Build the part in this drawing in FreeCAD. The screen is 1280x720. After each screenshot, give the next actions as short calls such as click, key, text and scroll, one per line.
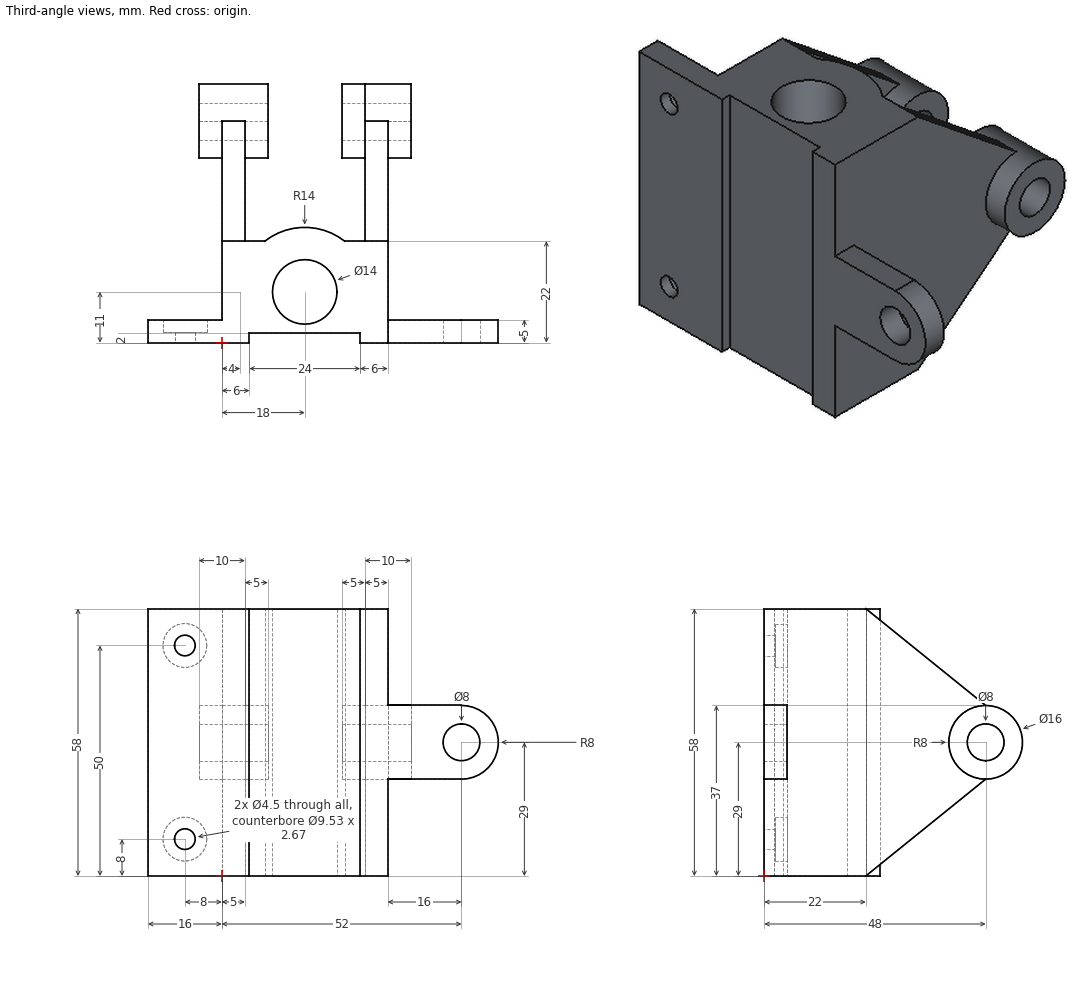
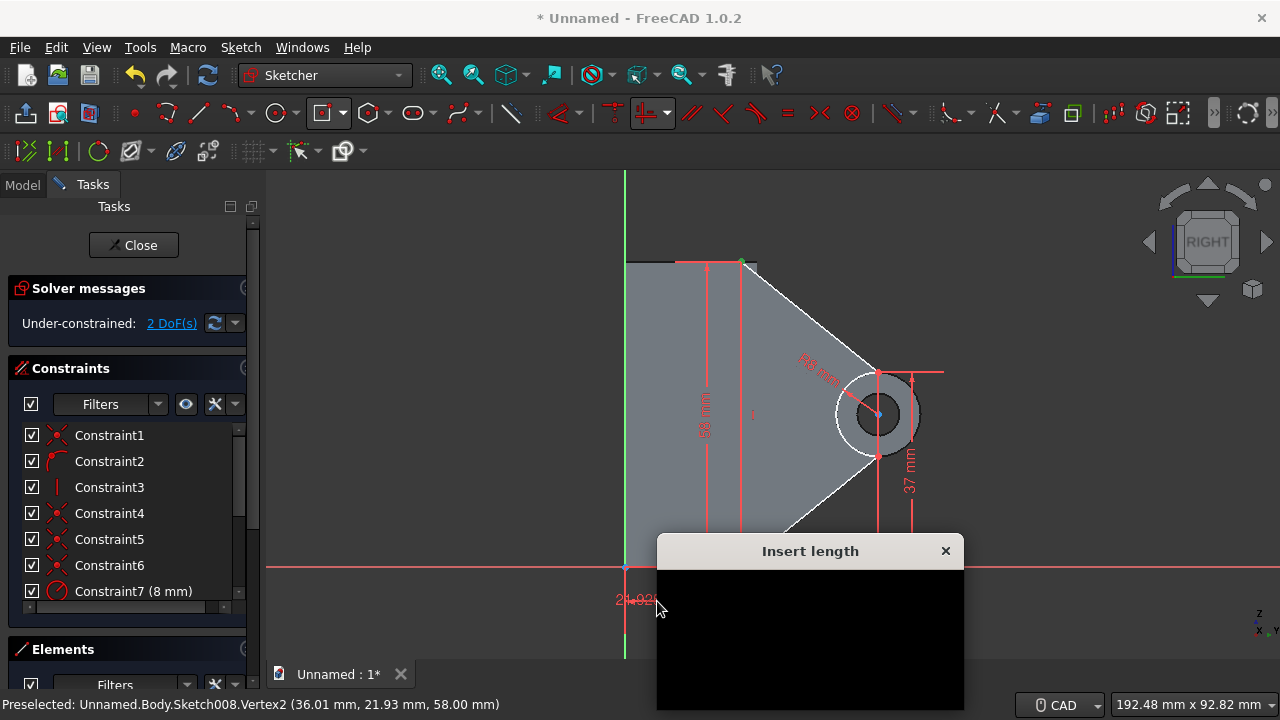
text(22)
key(Return)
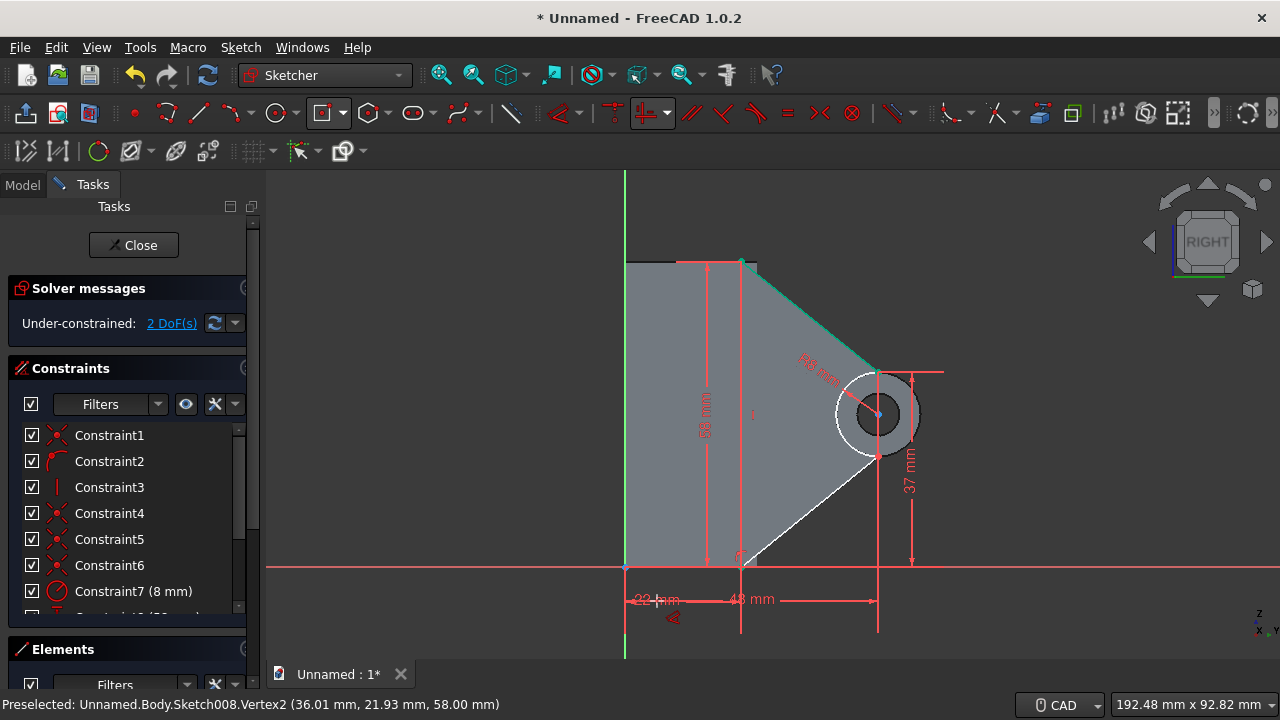
click(878, 457)
click(840, 601)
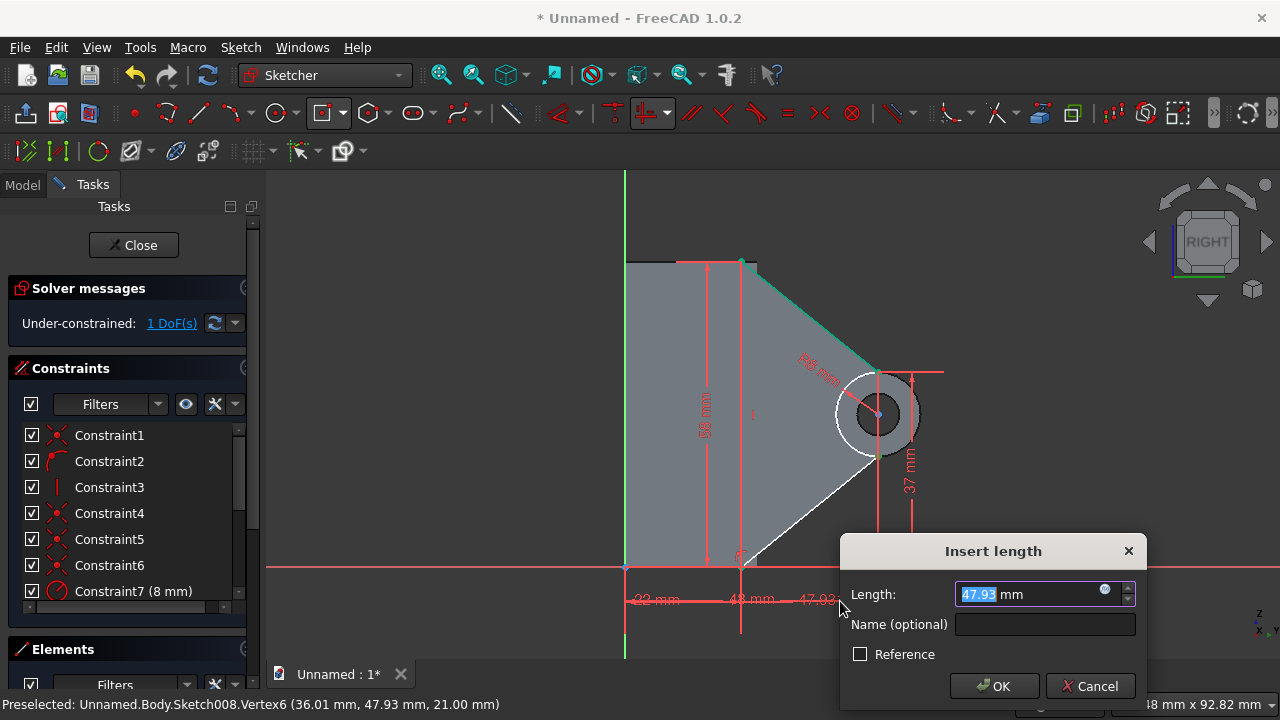
text(48)
key(Return)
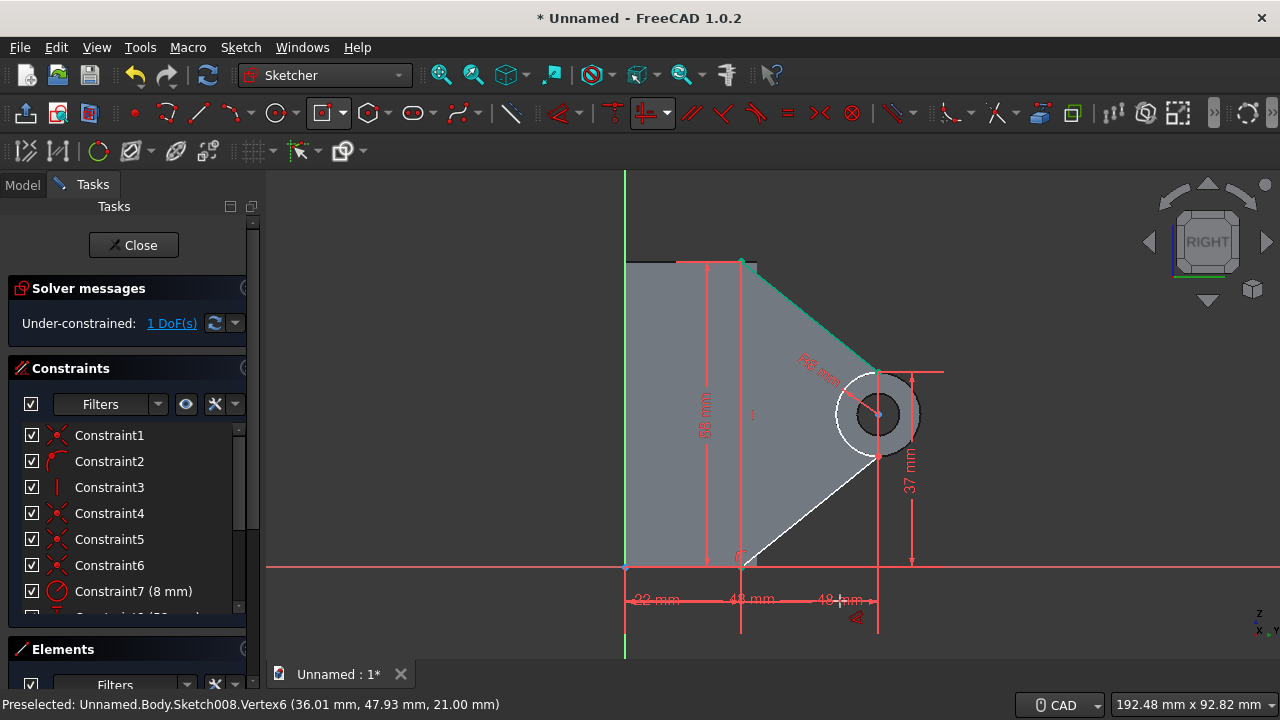
click(878, 414)
click(694, 380)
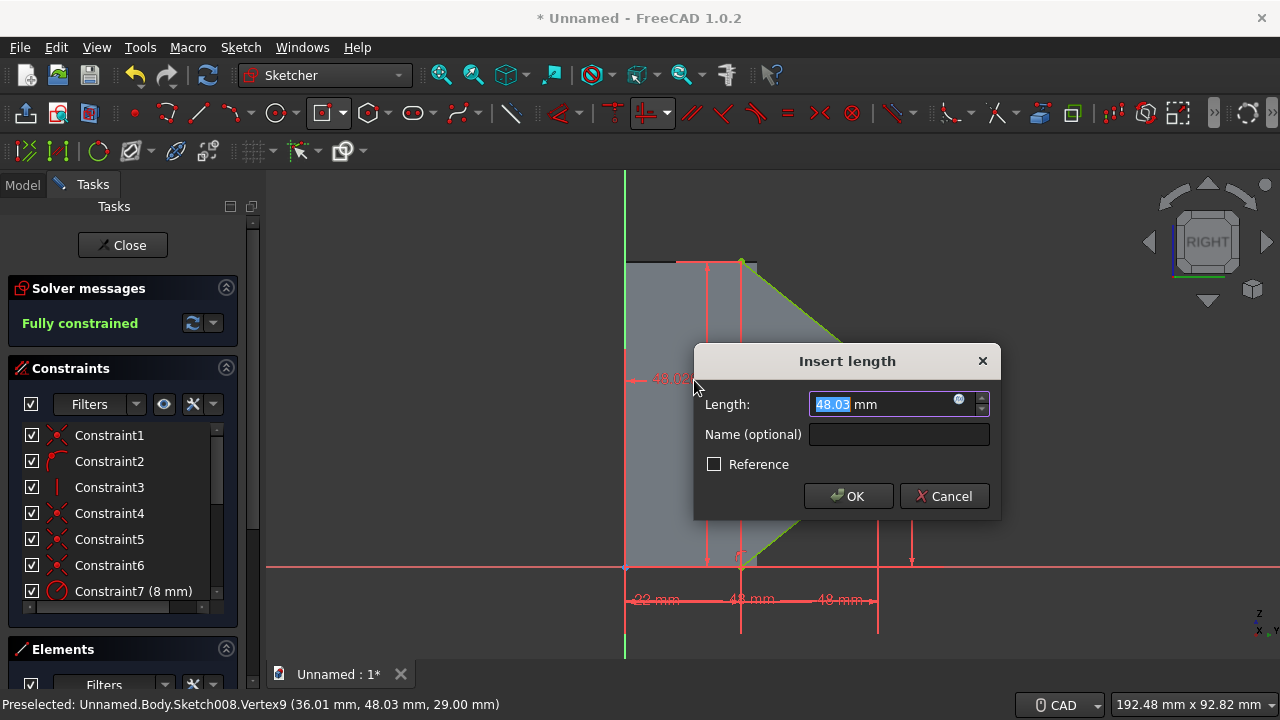
text(48)
key(Return)
key(Escape)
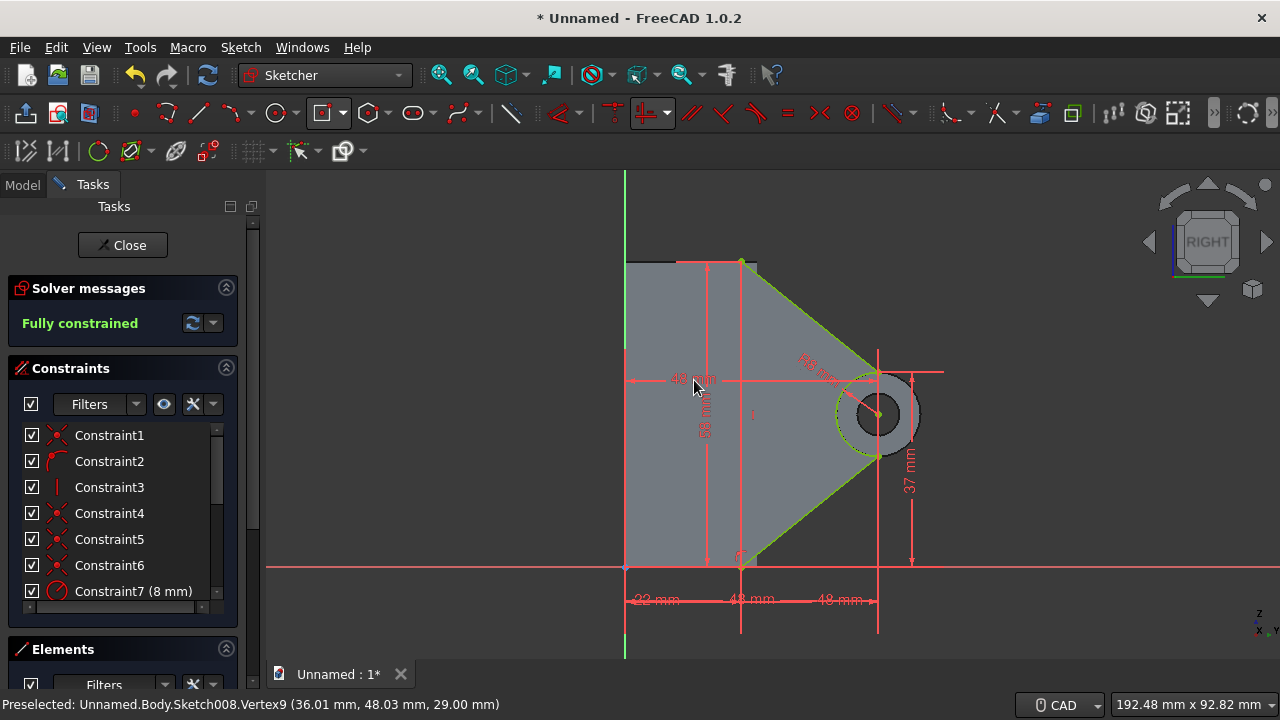
click(123, 245)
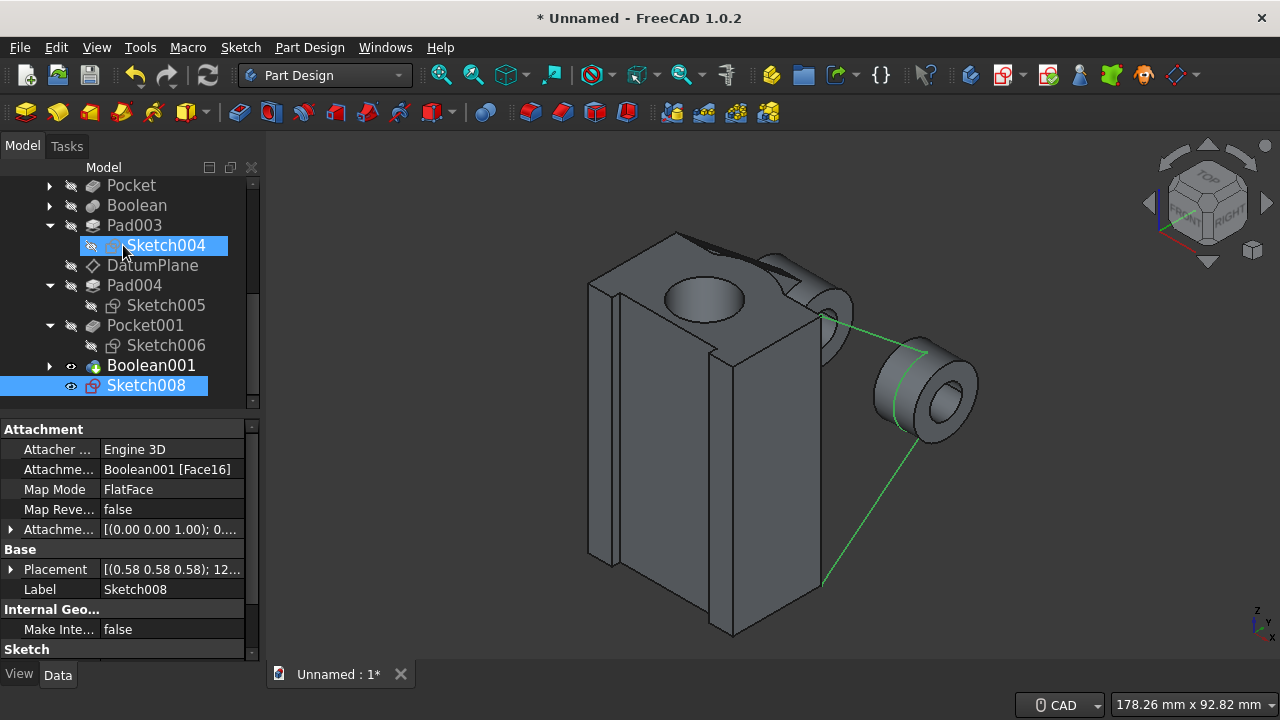
click(26, 112)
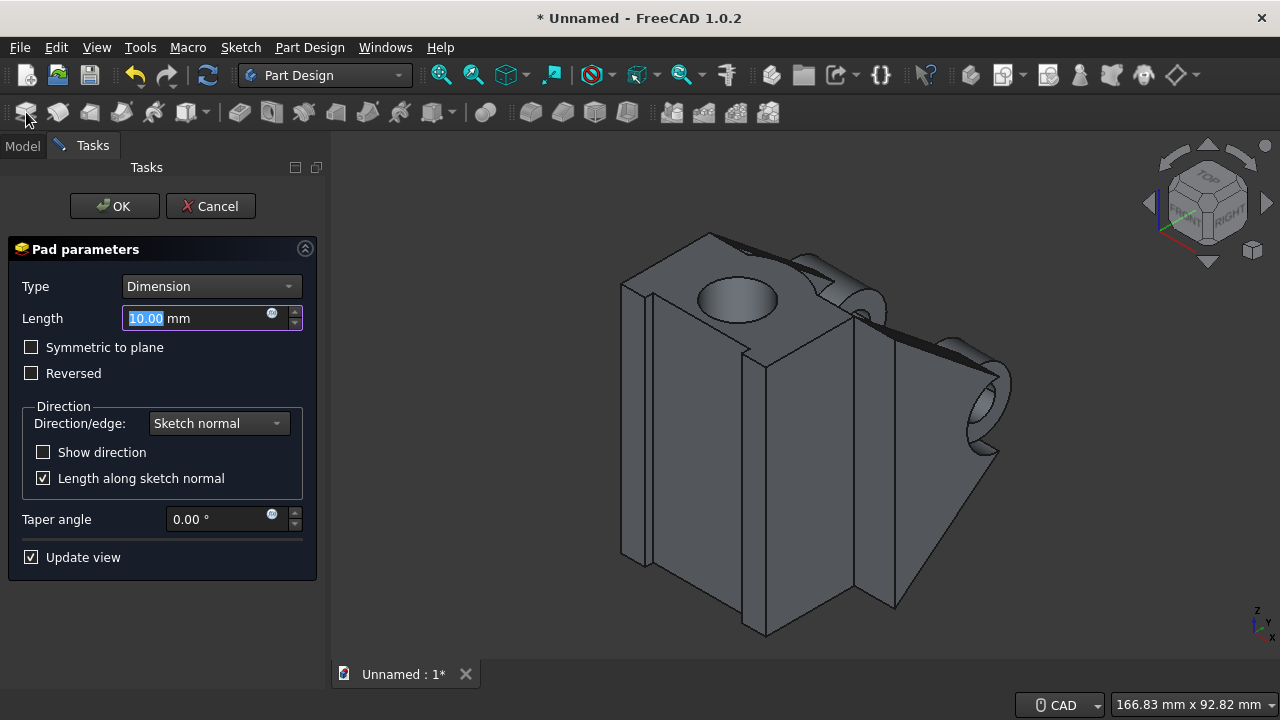
text(5)
key(Tab)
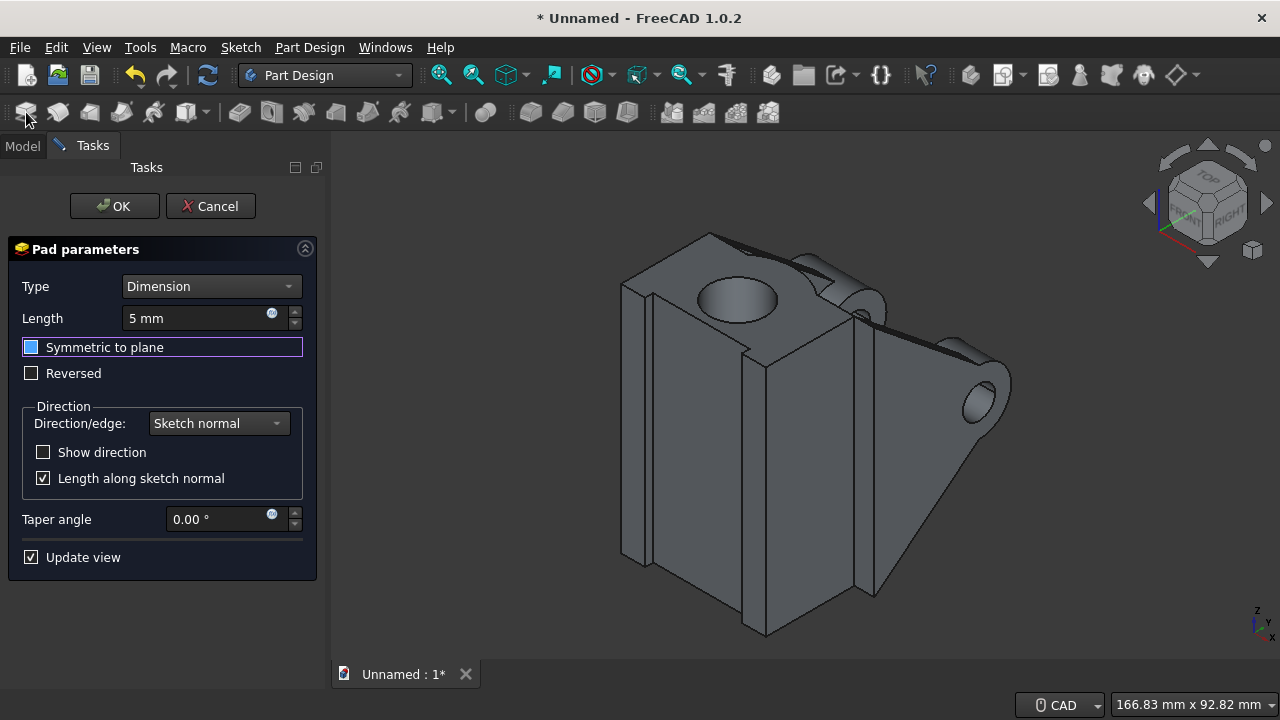
click(30, 373)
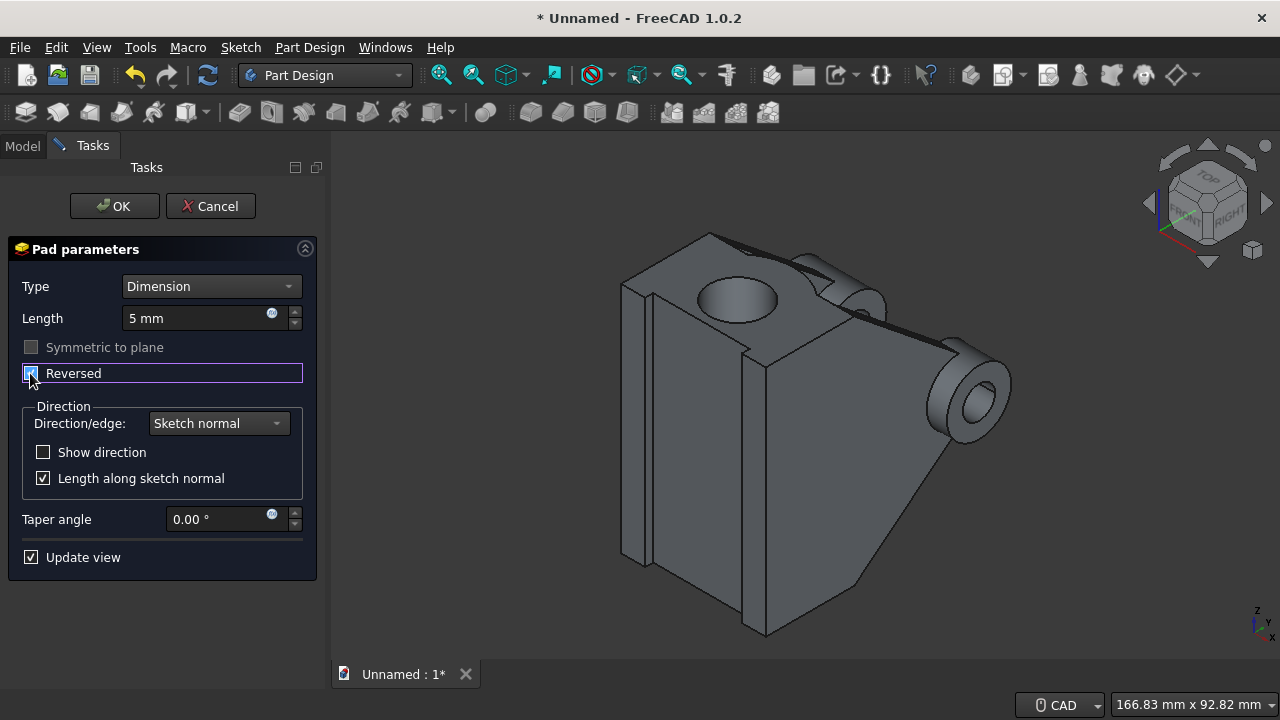
click(115, 206)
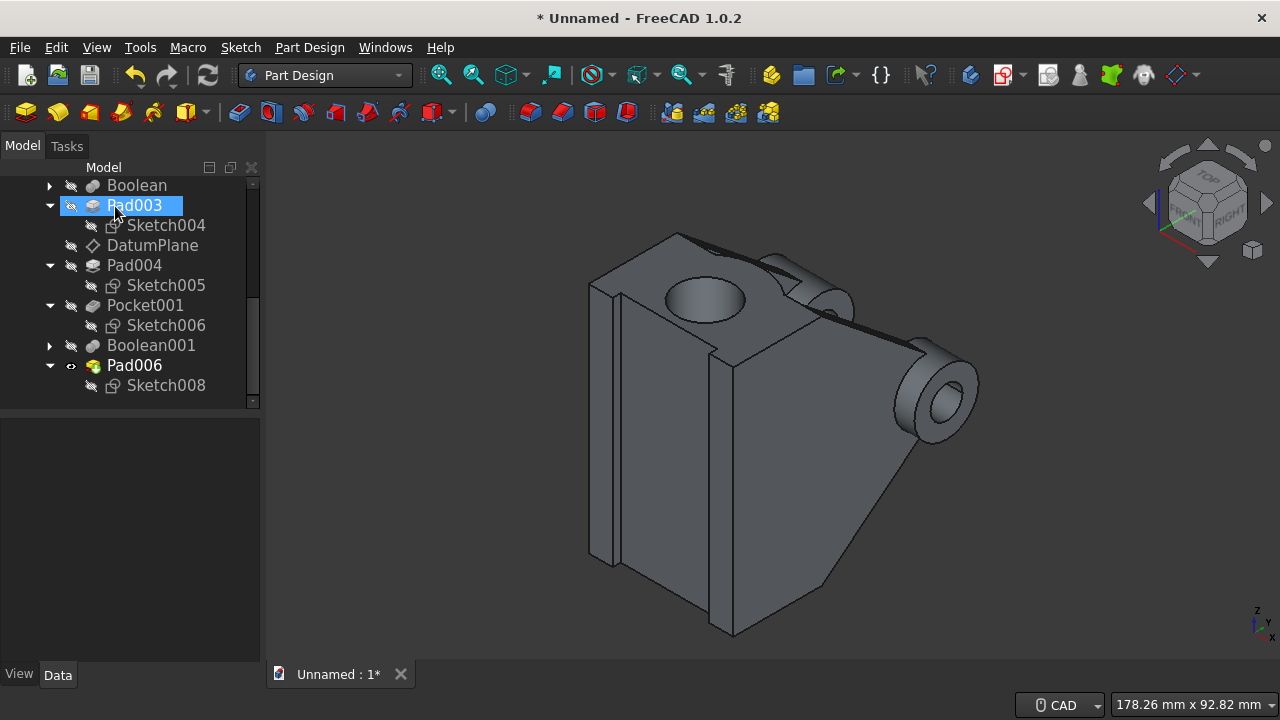
scroll(140, 281, down, 3)